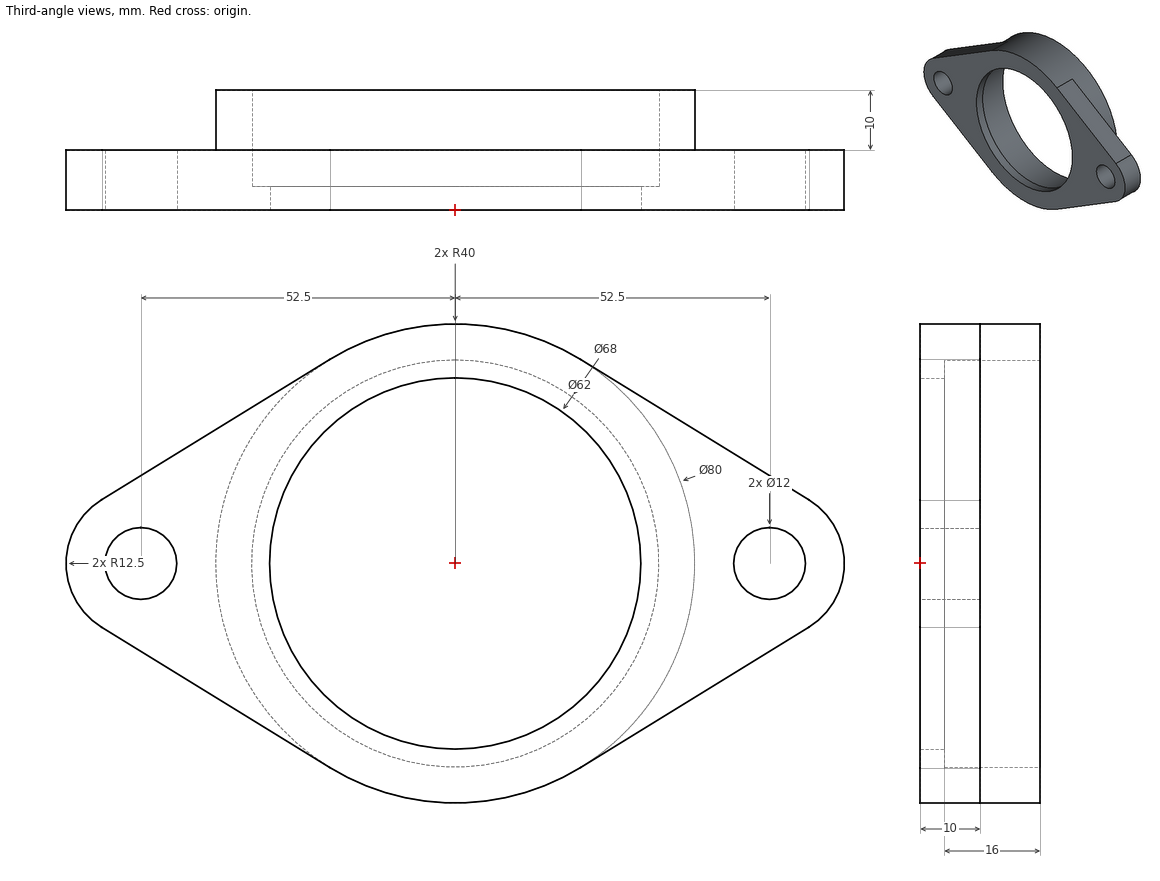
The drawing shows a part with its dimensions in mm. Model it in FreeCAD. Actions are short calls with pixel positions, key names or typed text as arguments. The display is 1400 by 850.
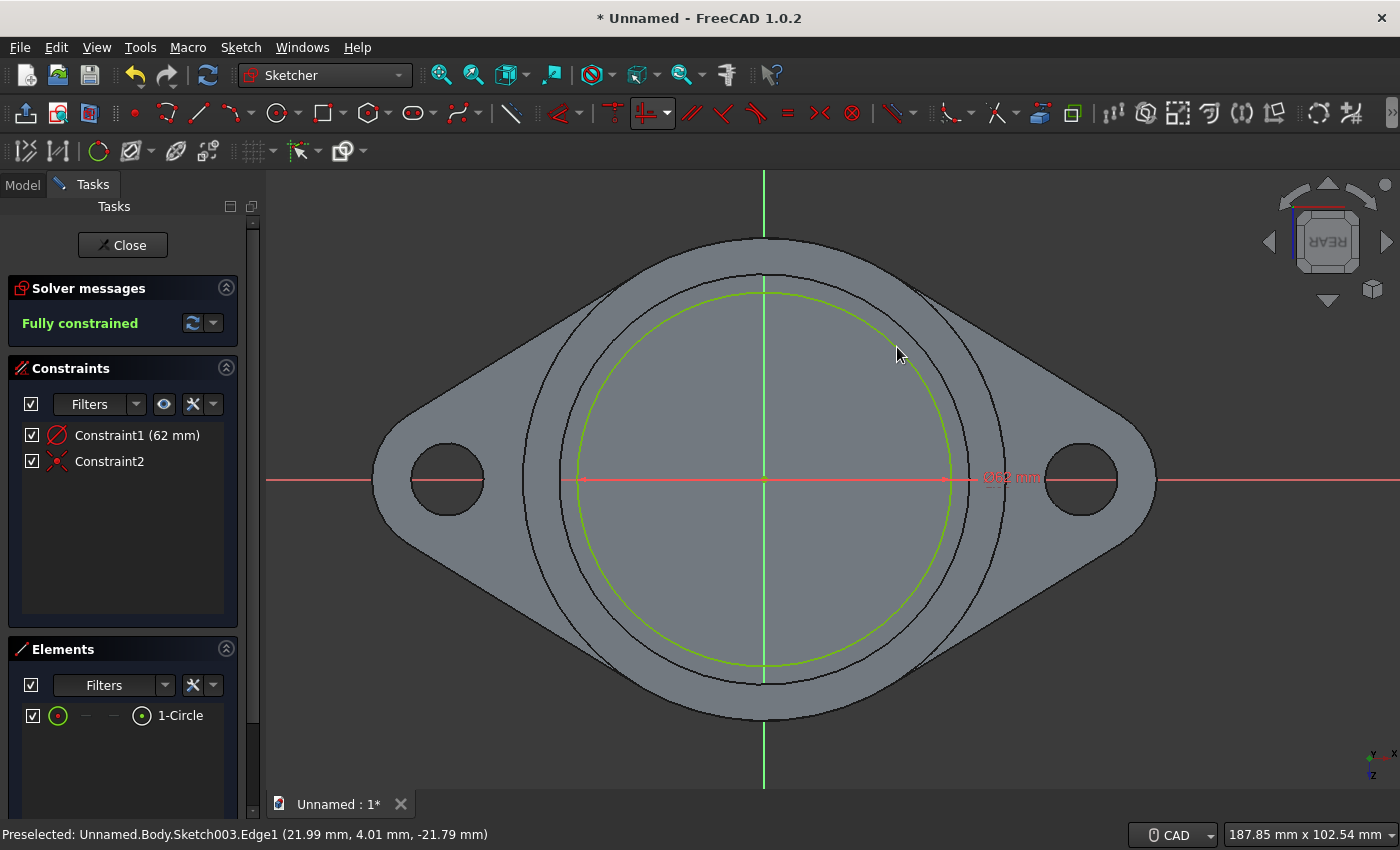
click(123, 245)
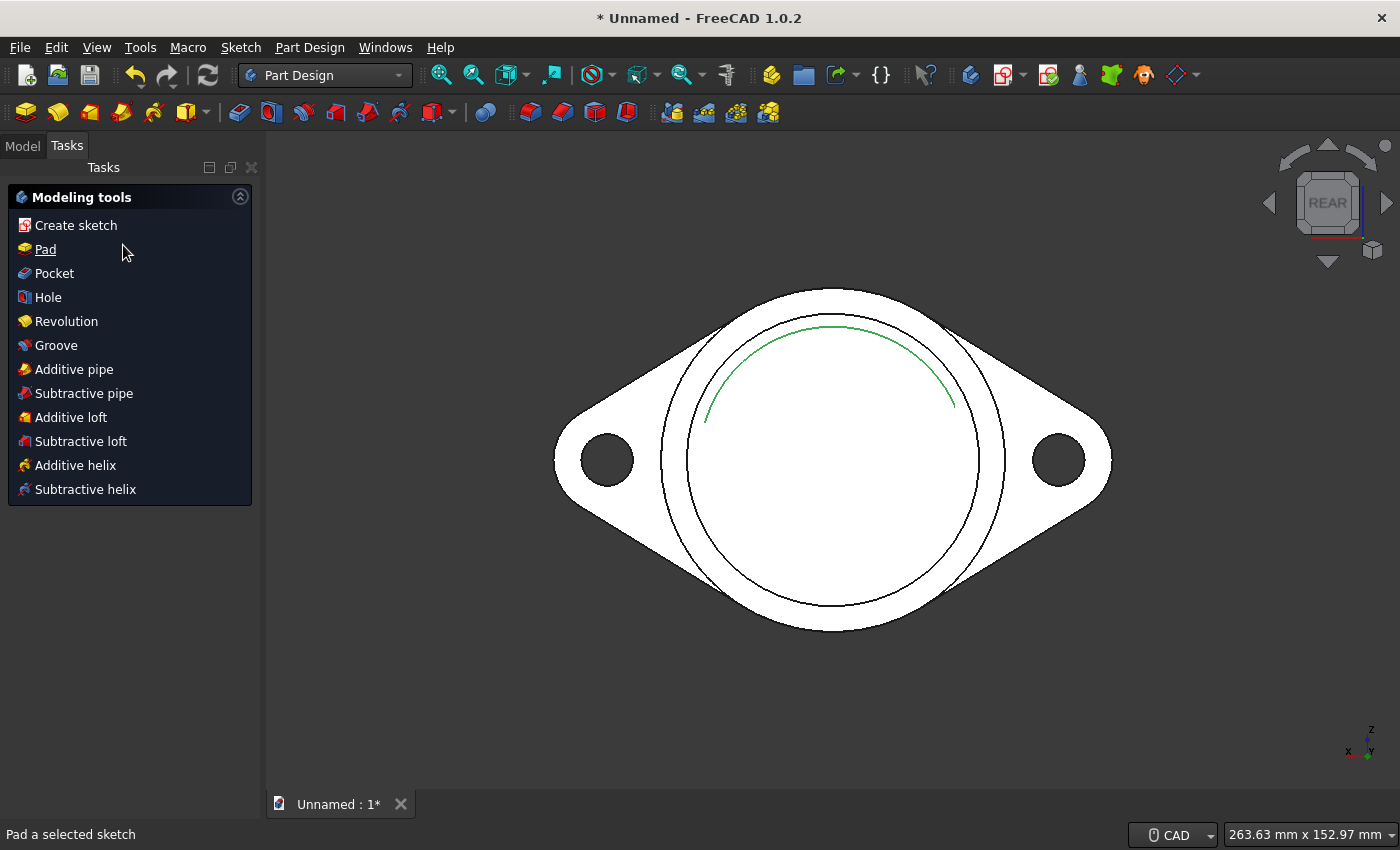
click(240, 112)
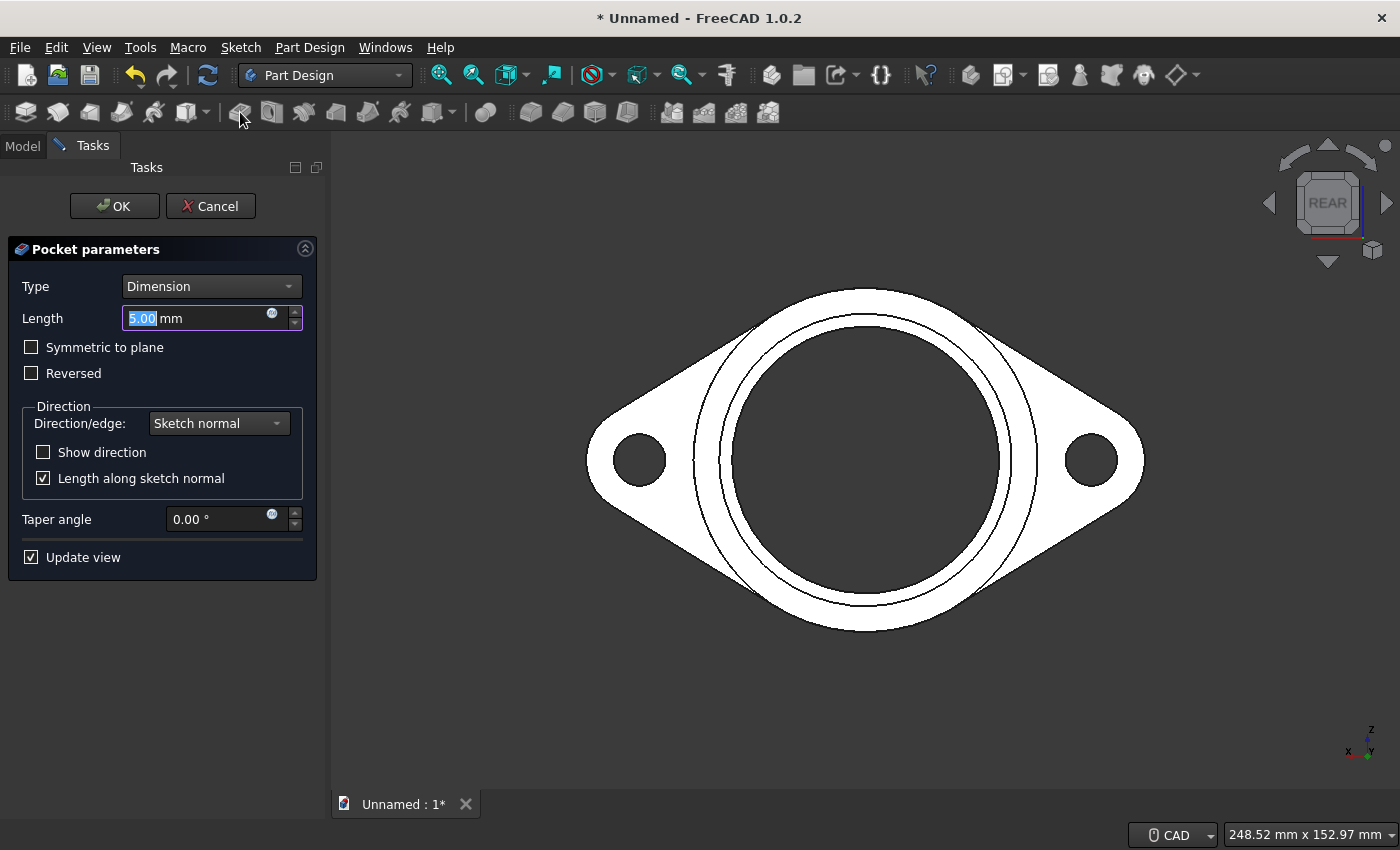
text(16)
key(Tab)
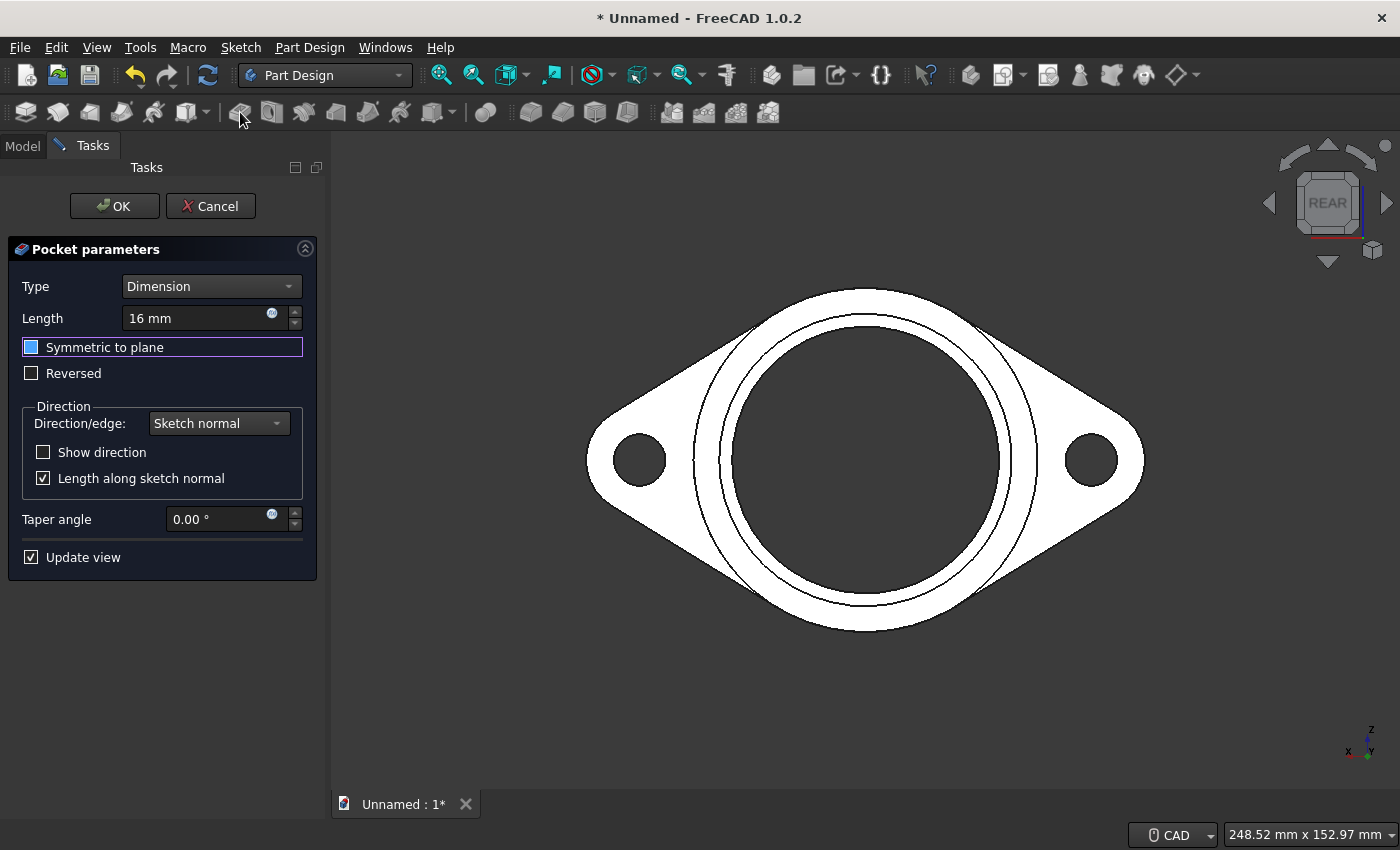
click(115, 206)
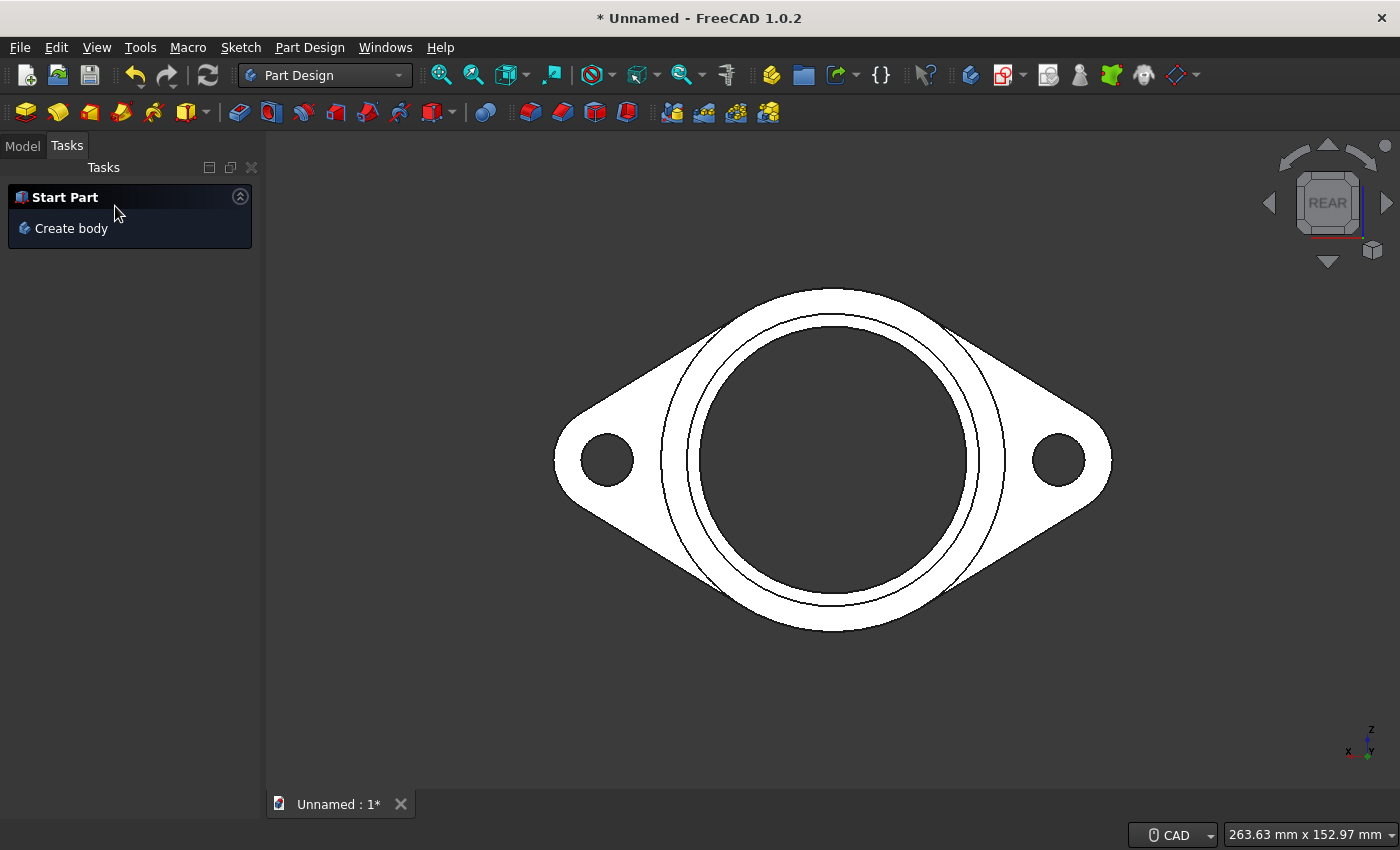
key(0)